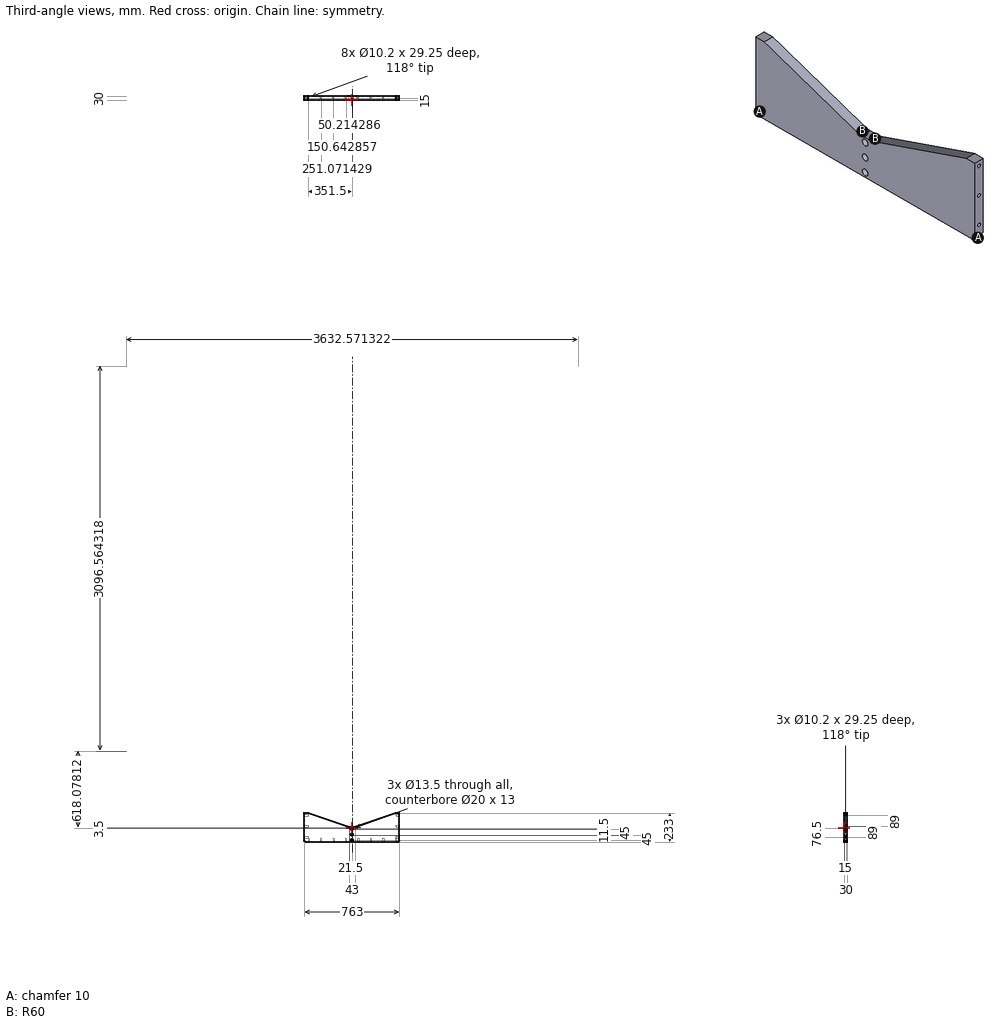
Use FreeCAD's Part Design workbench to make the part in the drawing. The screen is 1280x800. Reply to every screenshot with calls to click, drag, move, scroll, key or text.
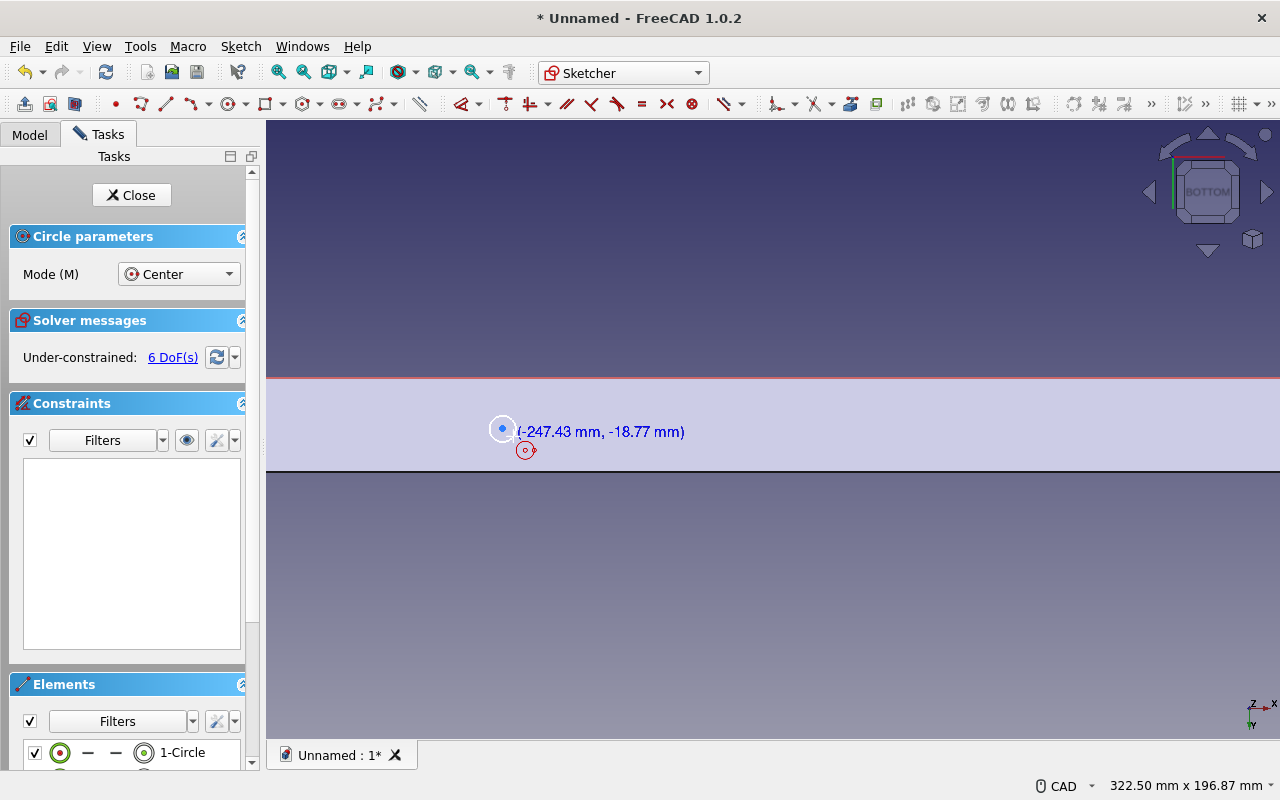
scroll(817, 425, up, 2)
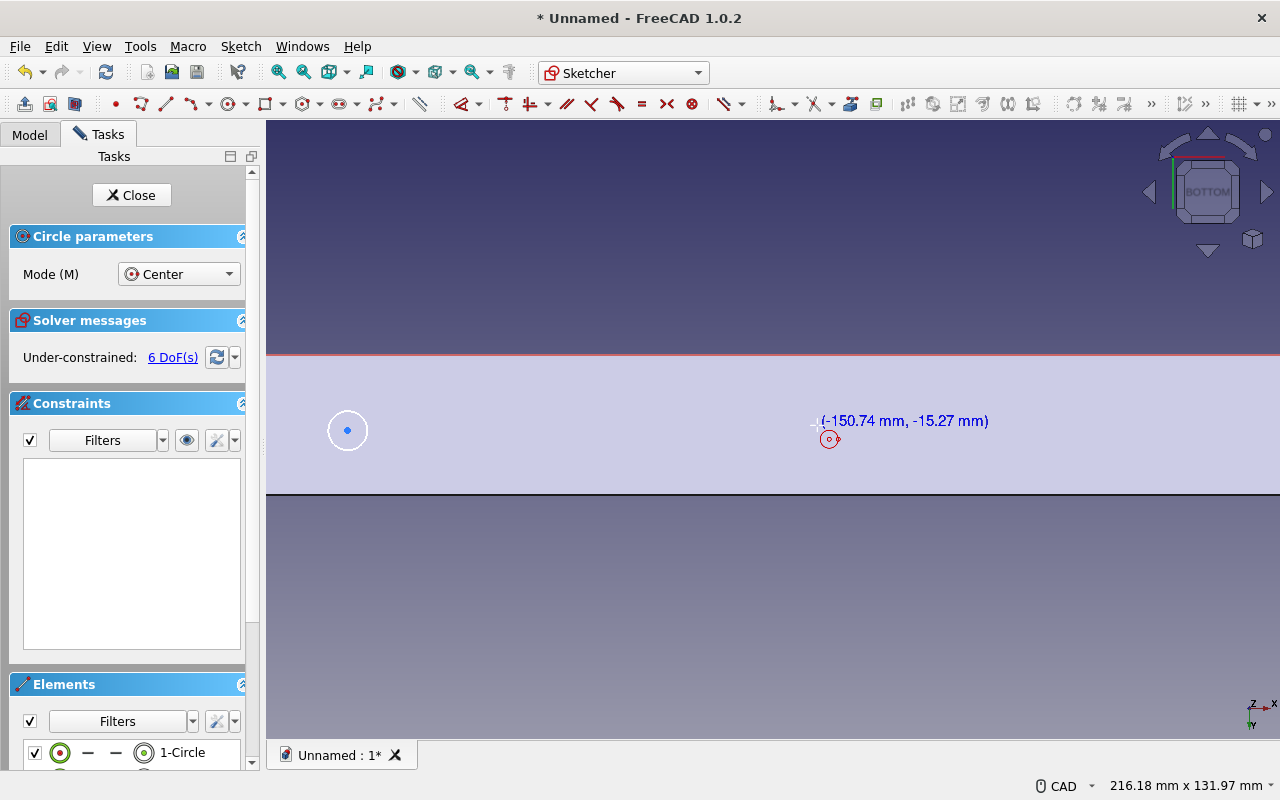
scroll(542, 435, down, 9)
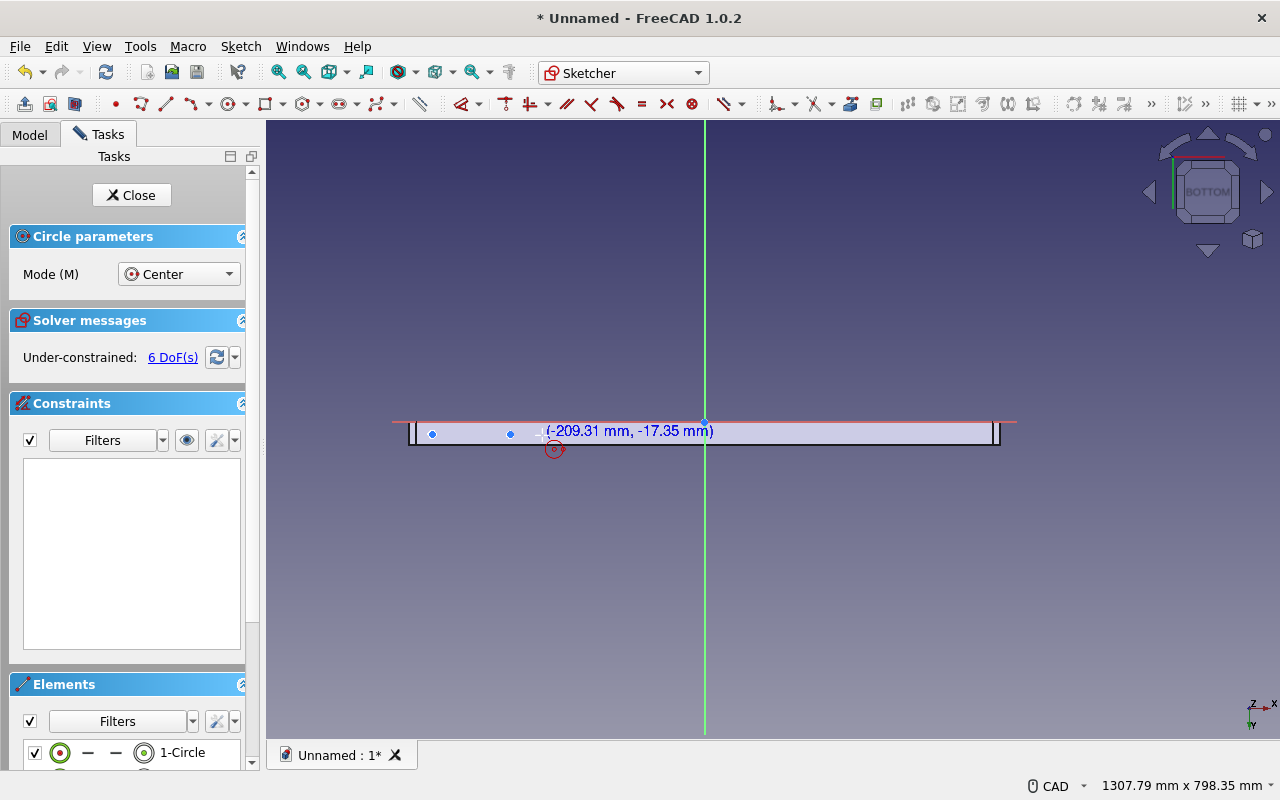
scroll(588, 434, up, 2)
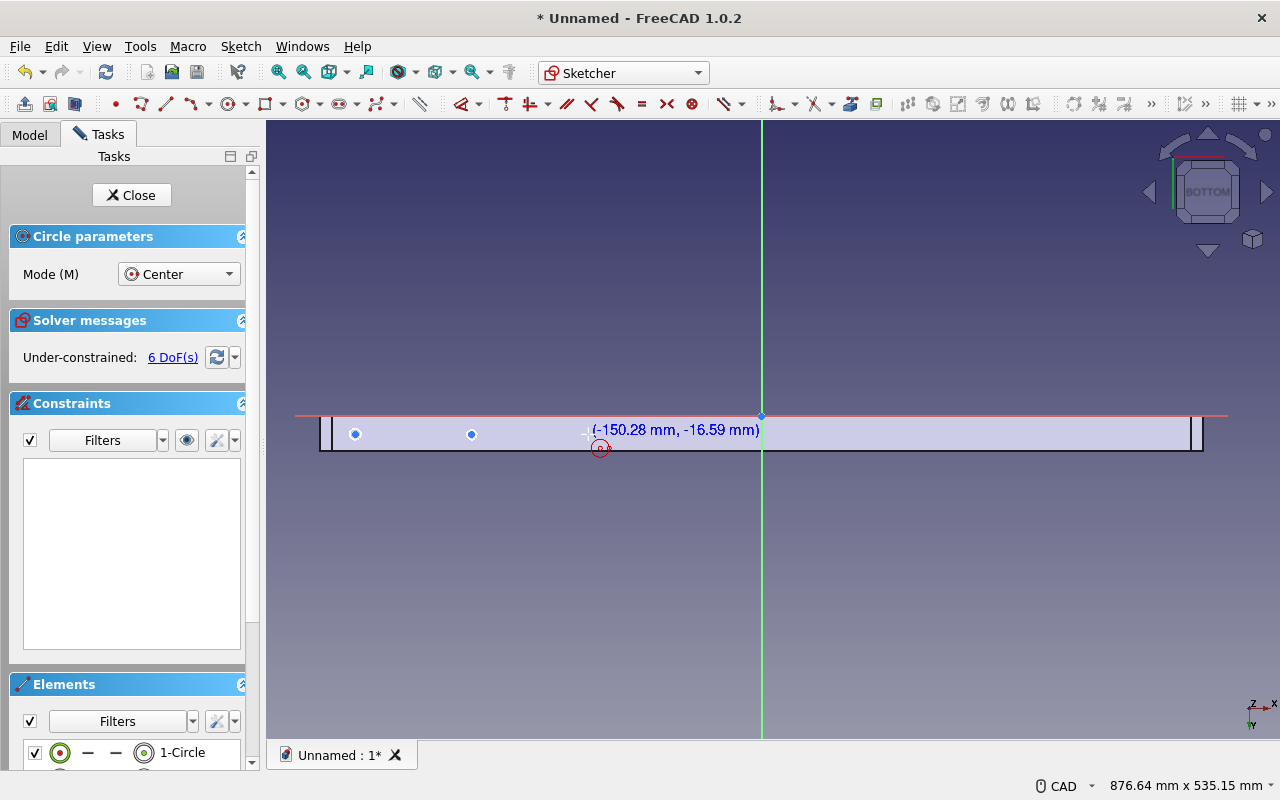
click(587, 433)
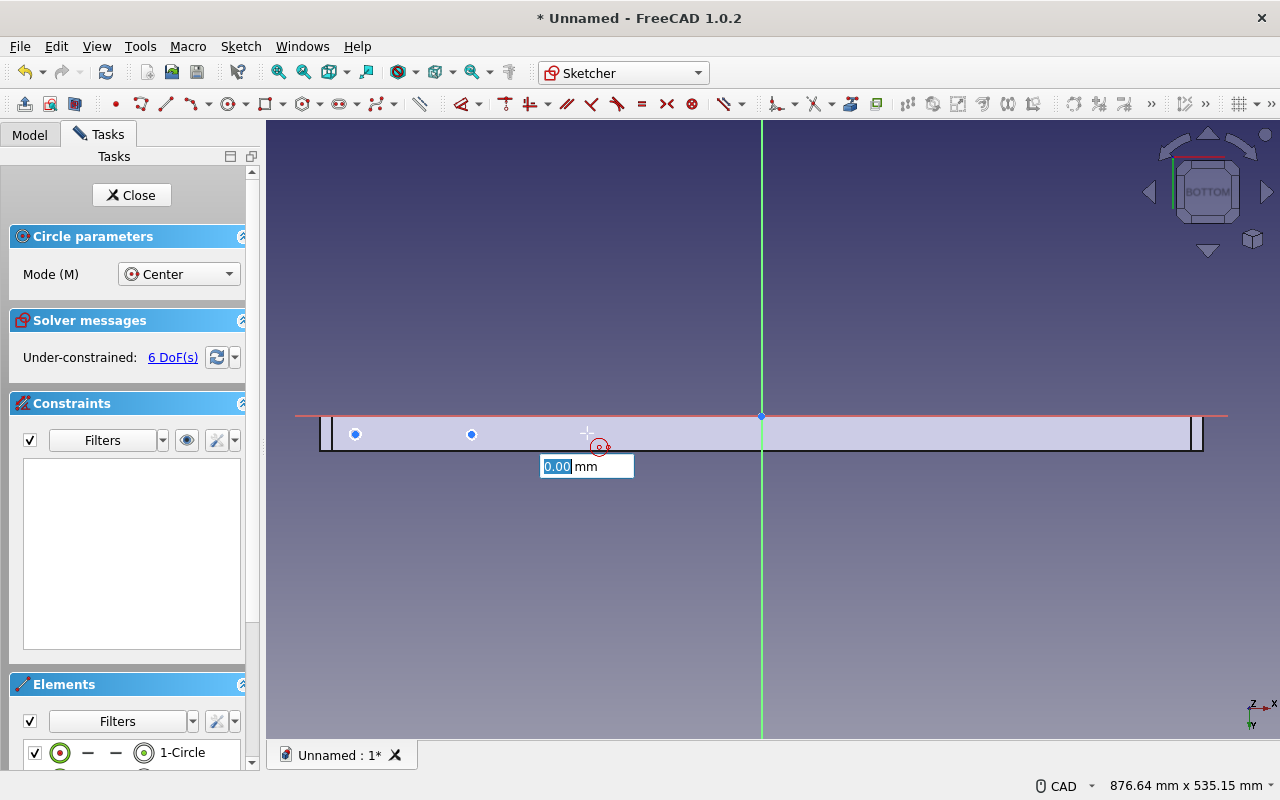
scroll(592, 438, up, 5)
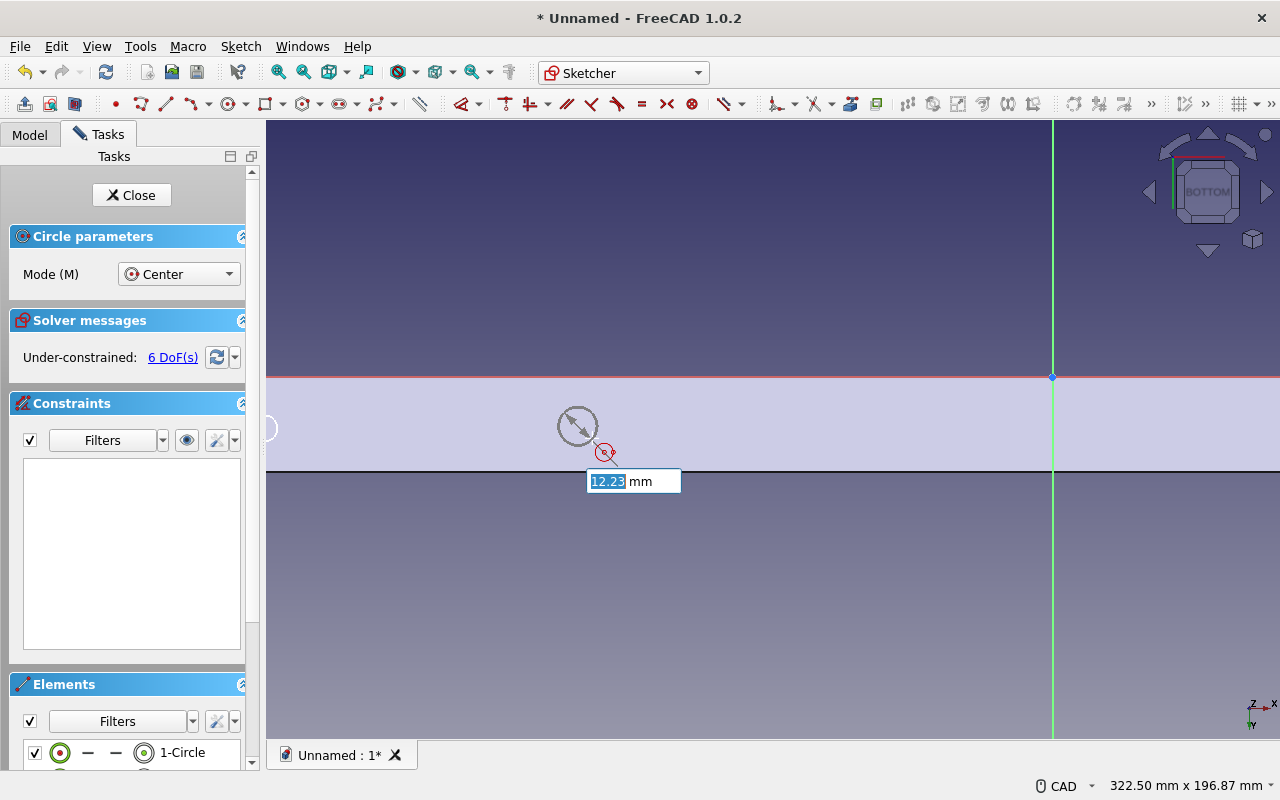
click(590, 436)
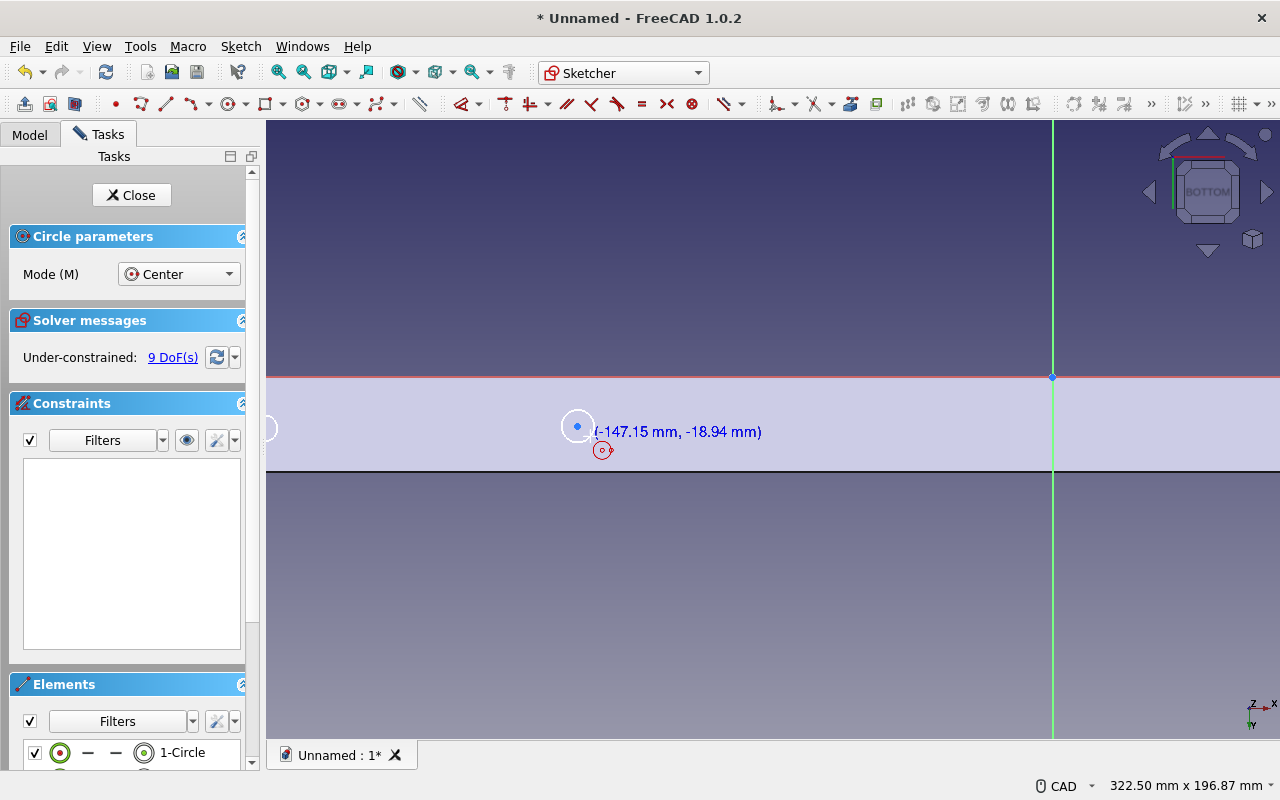
scroll(895, 425, up, 2)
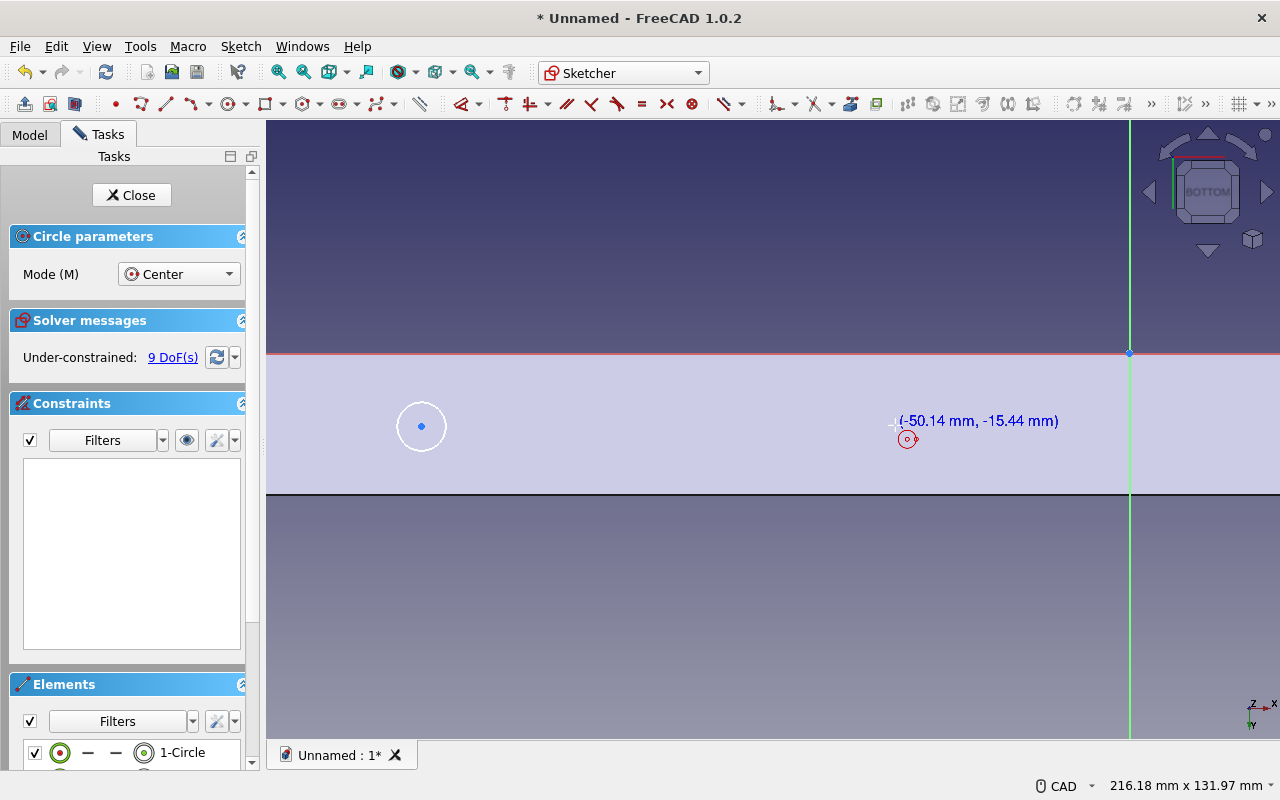
scroll(620, 435, down, 9)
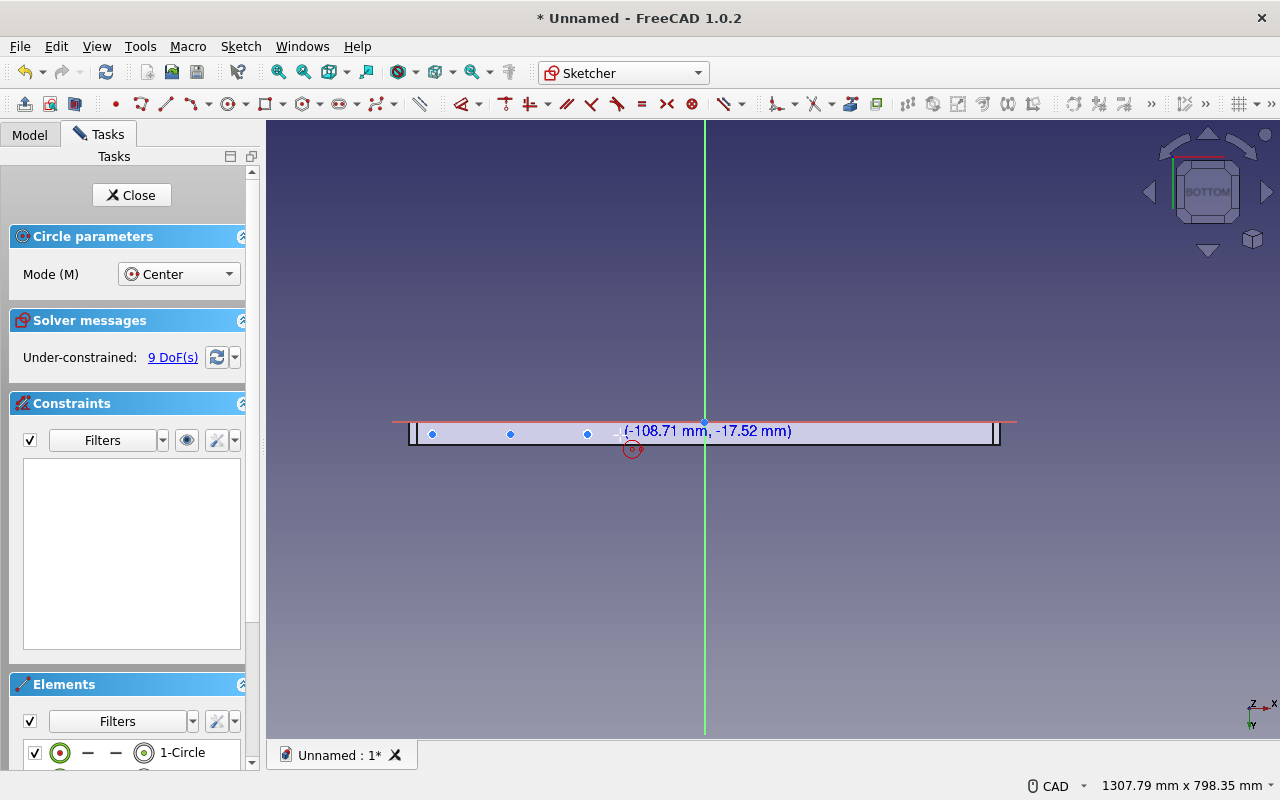
scroll(666, 434, up, 2)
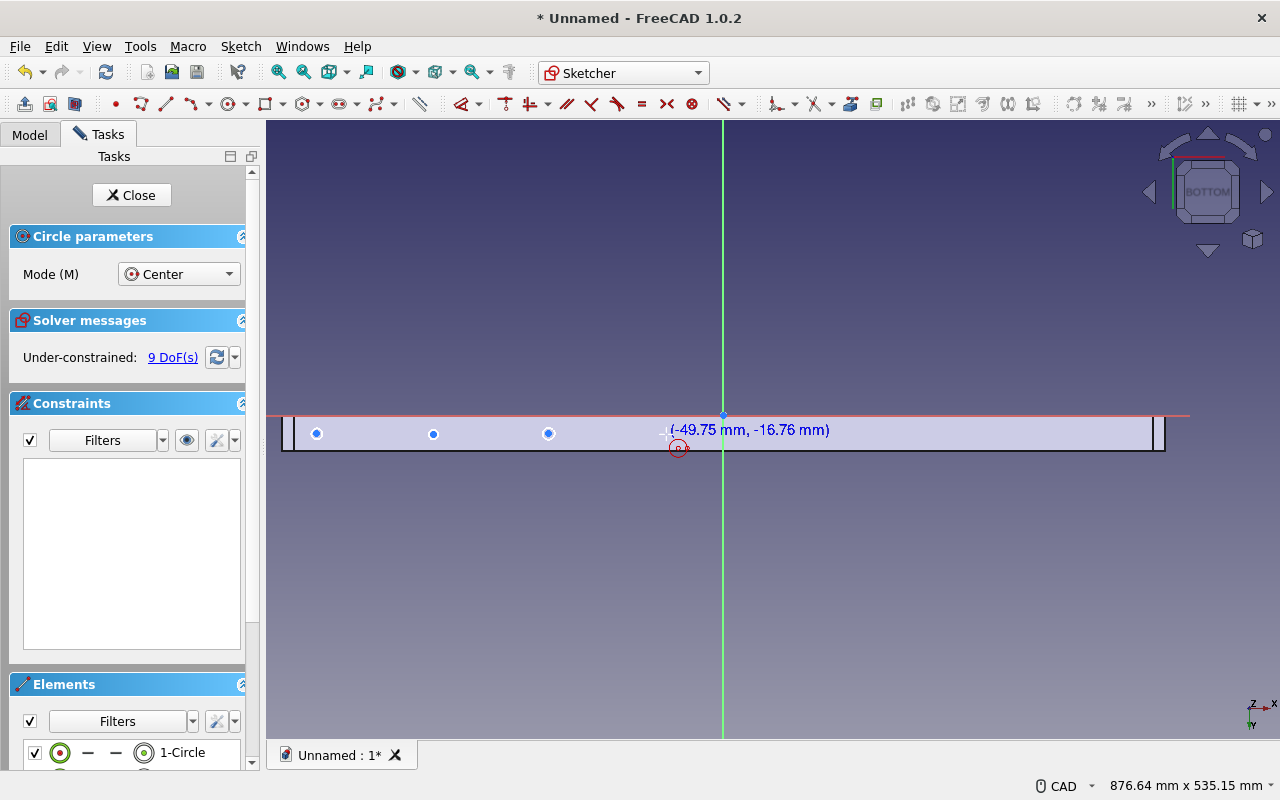
click(665, 433)